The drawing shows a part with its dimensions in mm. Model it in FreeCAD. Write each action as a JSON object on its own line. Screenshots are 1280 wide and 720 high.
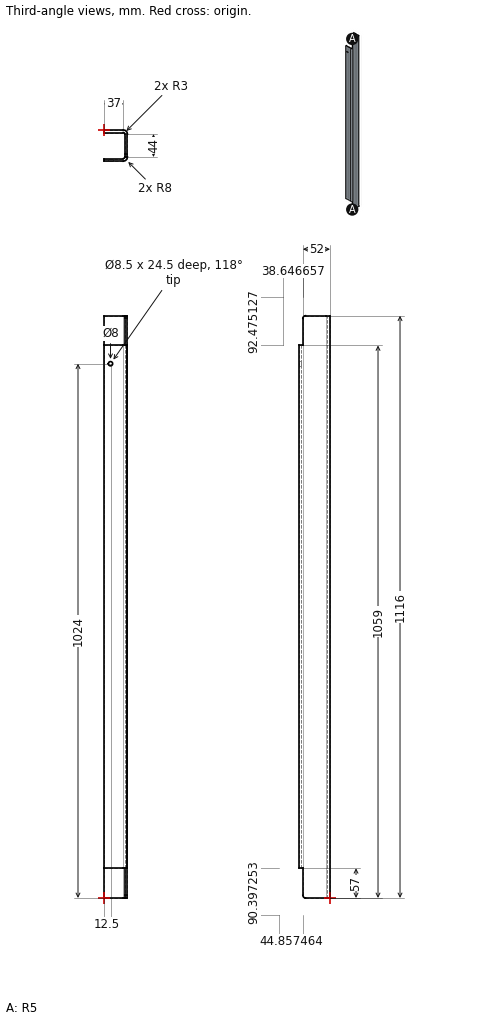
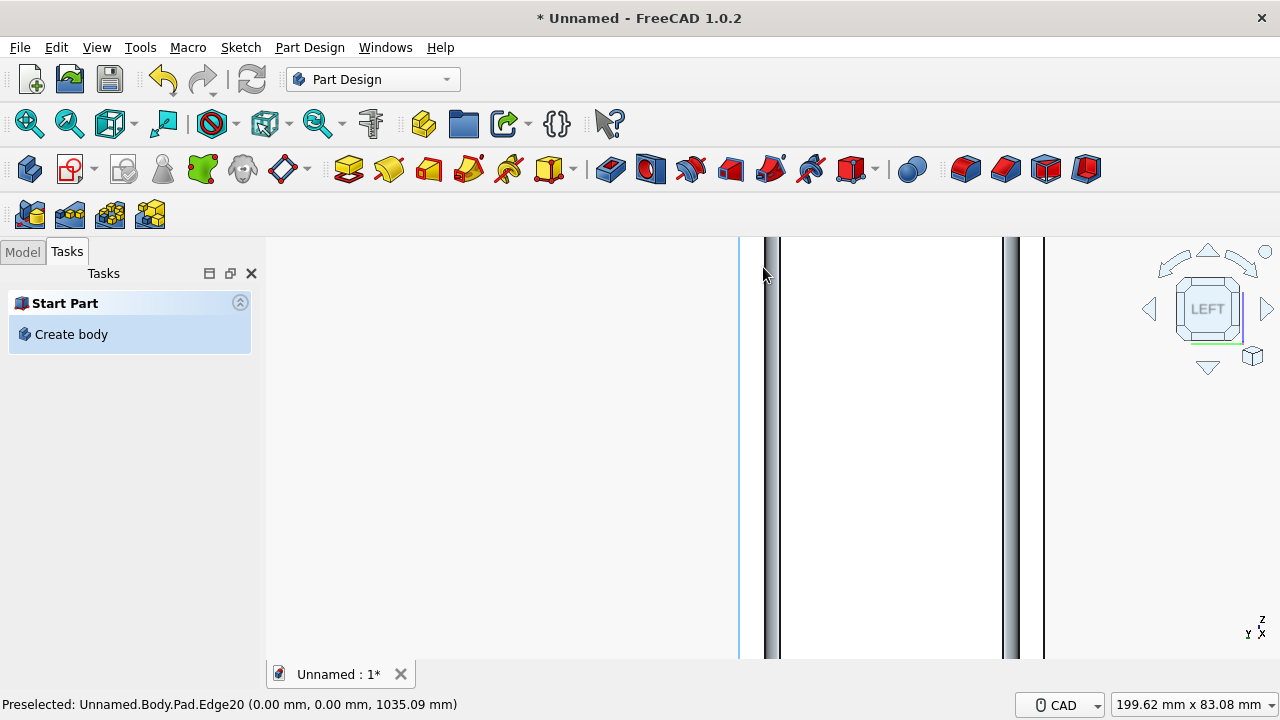
{"action": "left_click", "coordinate": [752, 273]}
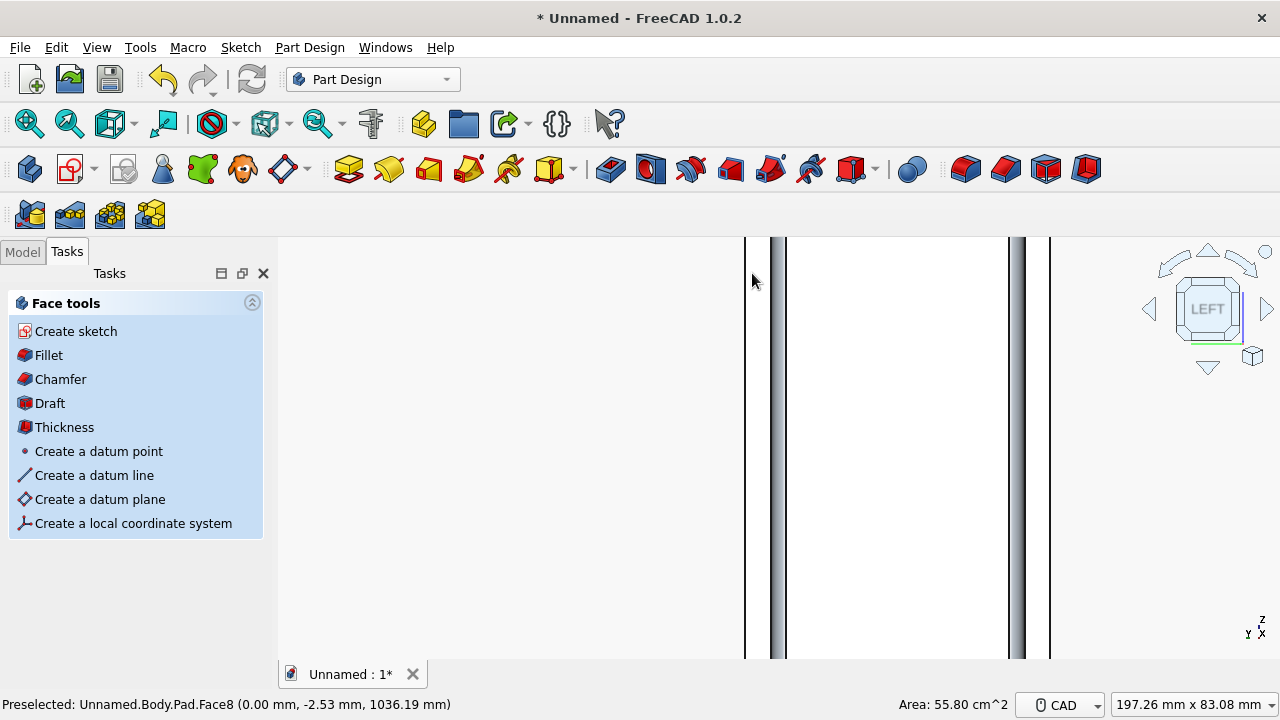
{"action": "left_click", "coordinate": [70, 170]}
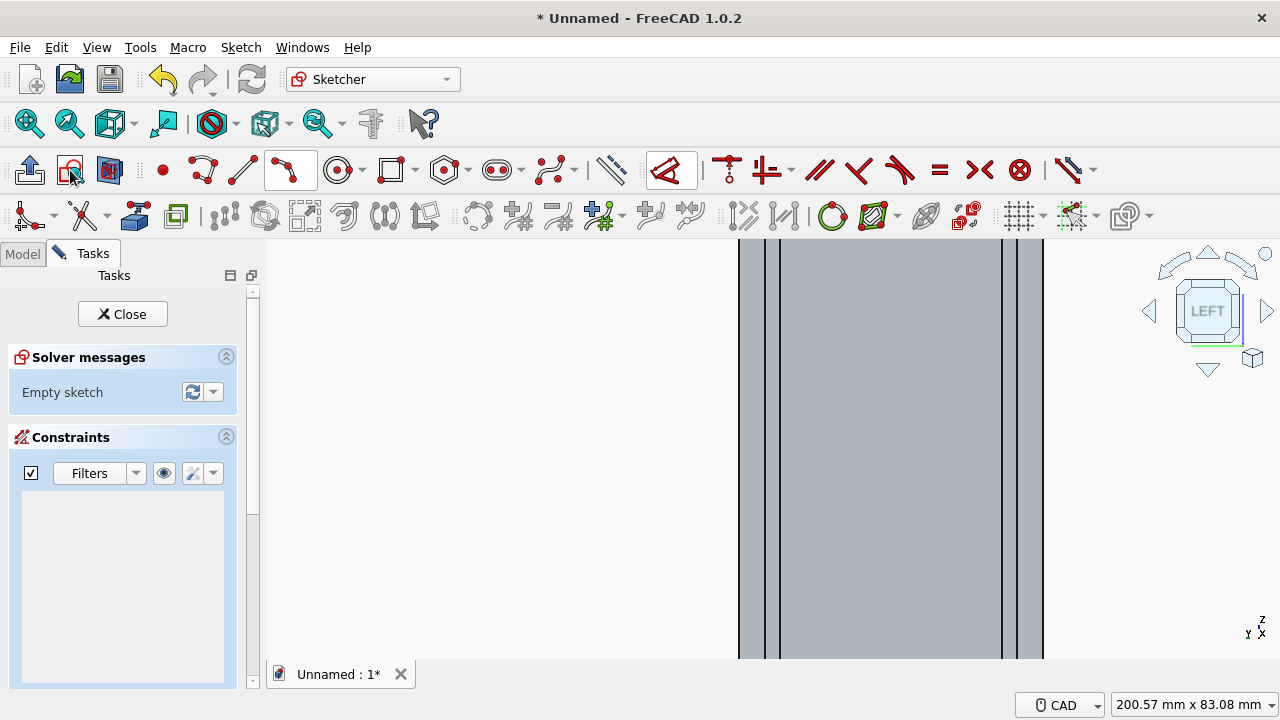
{"action": "scroll", "coordinate": [690, 332], "scroll_direction": "down", "scroll_amount": 15}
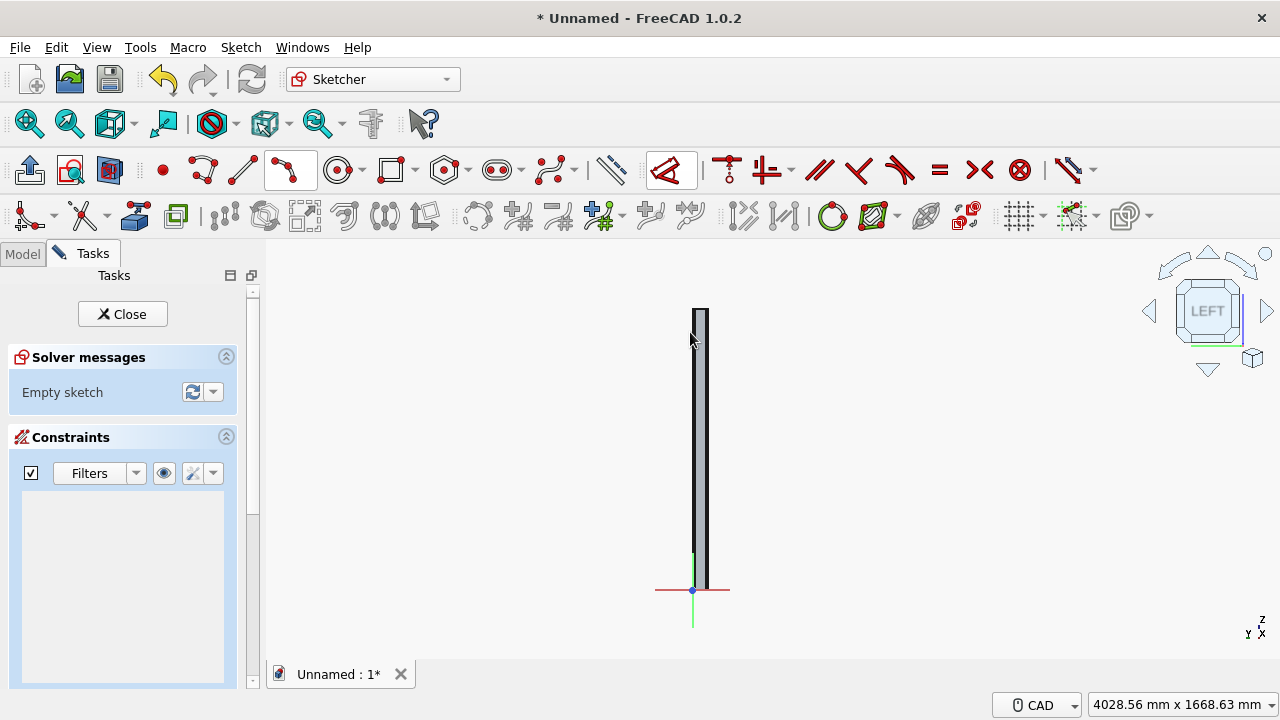
{"action": "left_click", "coordinate": [392, 170]}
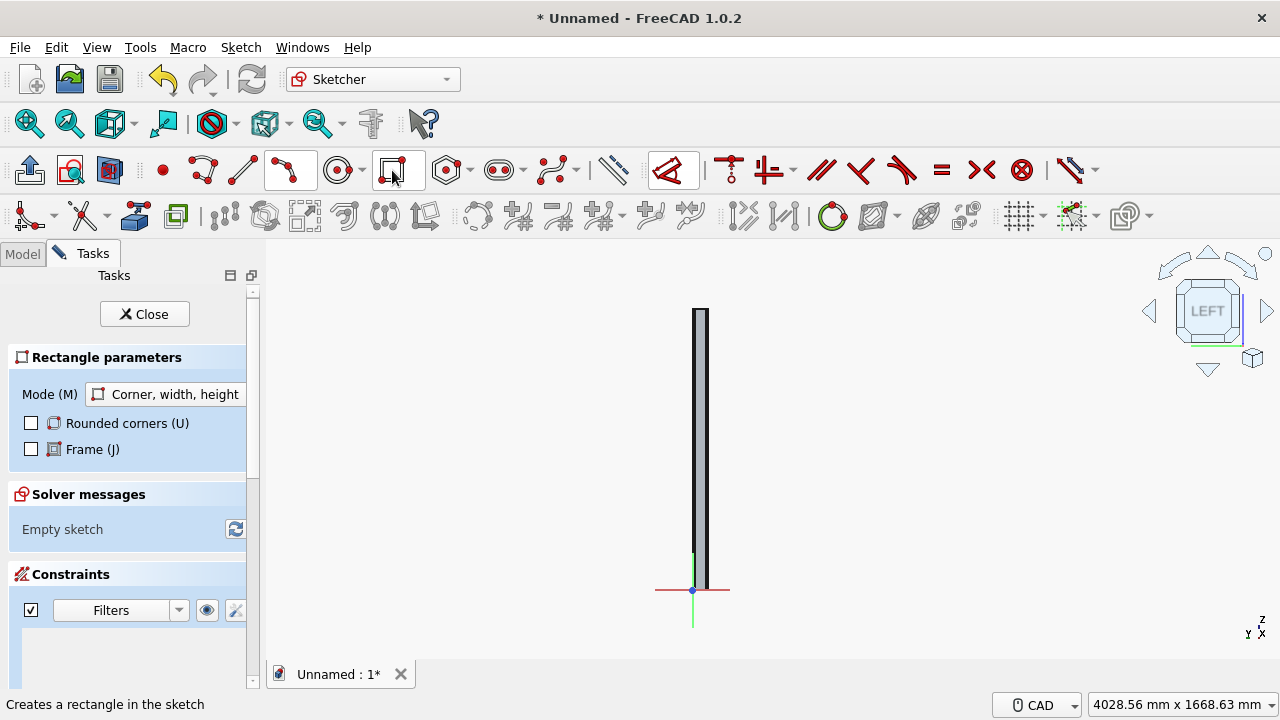
{"action": "scroll", "coordinate": [706, 300], "scroll_direction": "up", "scroll_amount": 3}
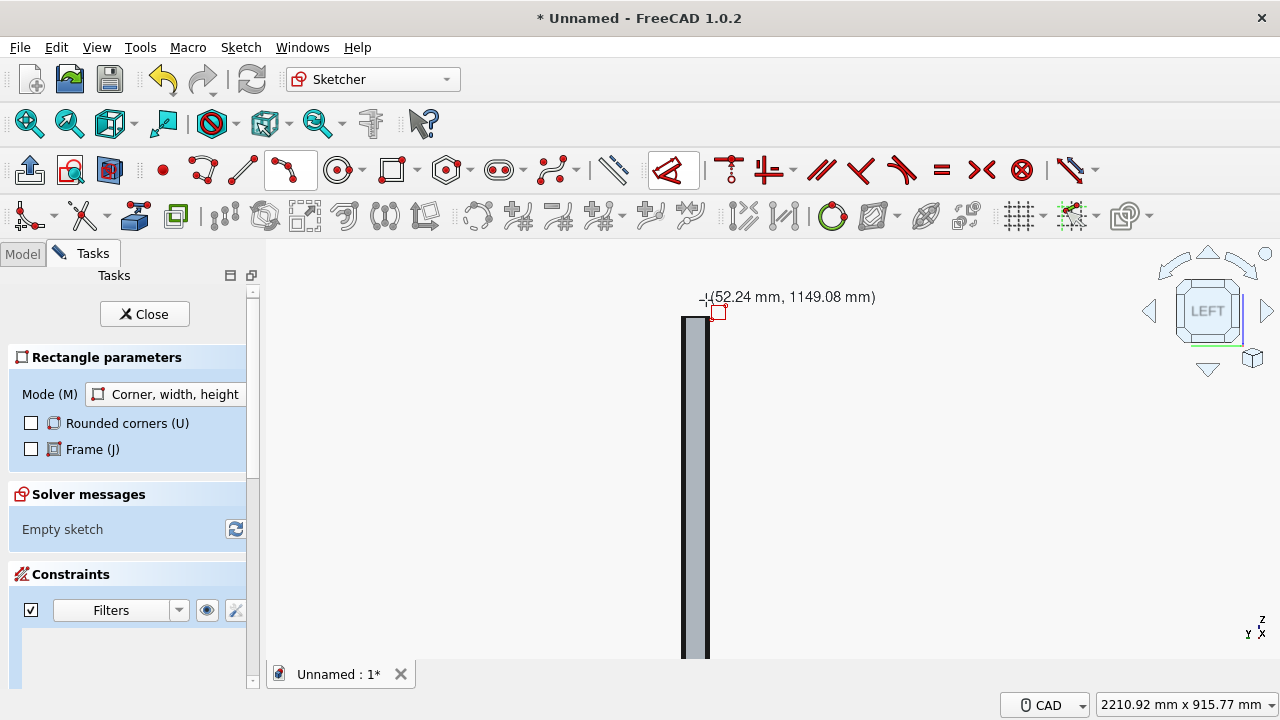
{"action": "left_click", "coordinate": [706, 301]}
{"action": "mouse_move", "coordinate": [723, 343]}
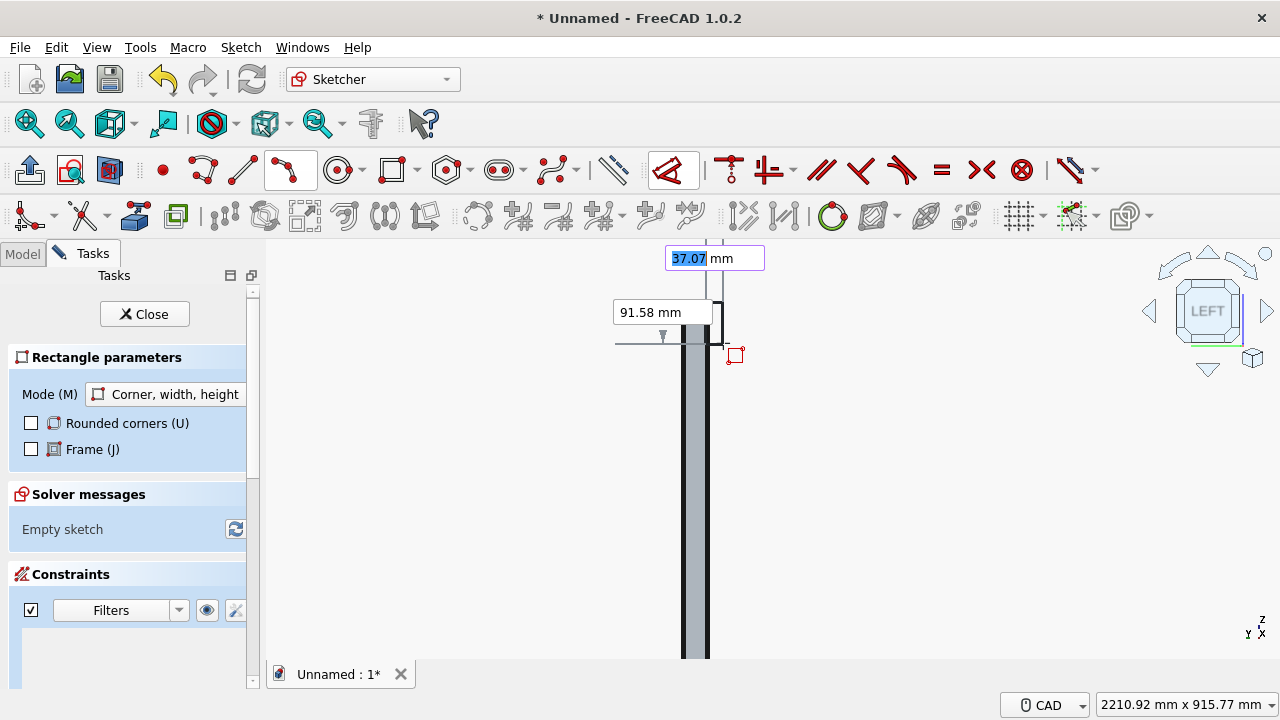
{"action": "type", "text": "38.646657"}
{"action": "key", "text": "Tab"}
{"action": "type", "text": "92.475127"}
{"action": "key", "text": "Return"}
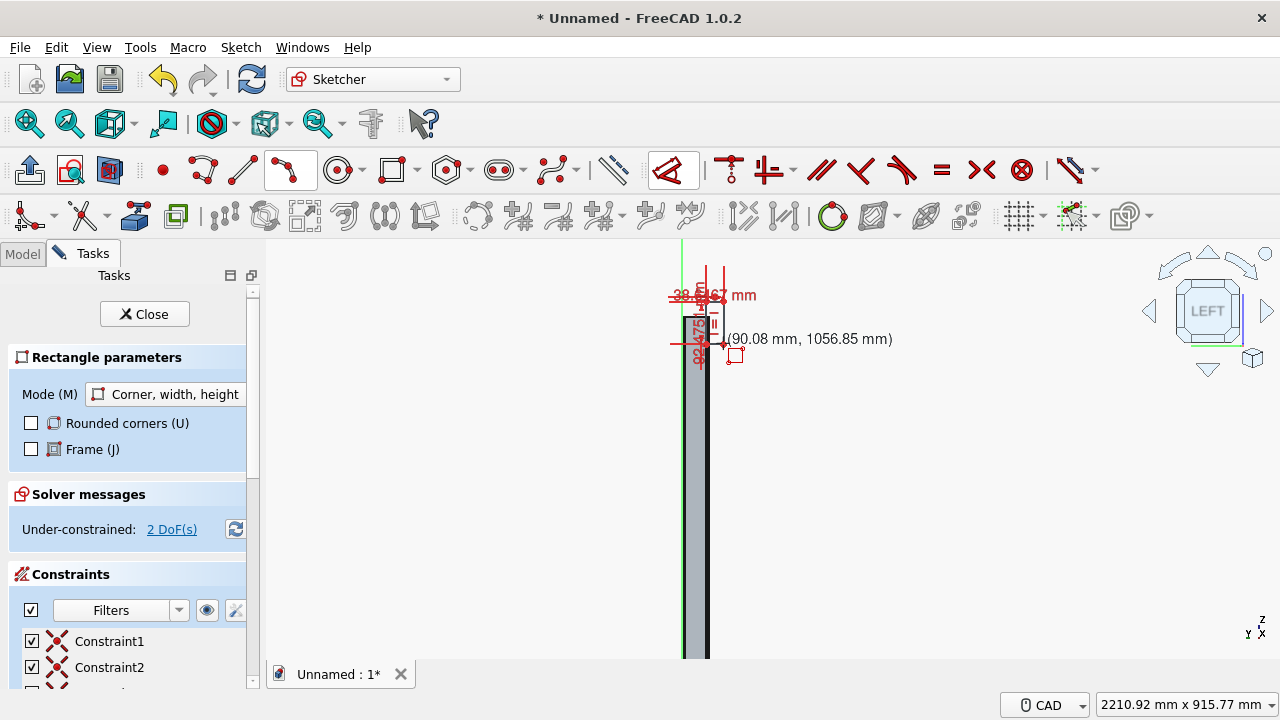
{"action": "scroll", "coordinate": [705, 348], "scroll_direction": "down", "scroll_amount": 4}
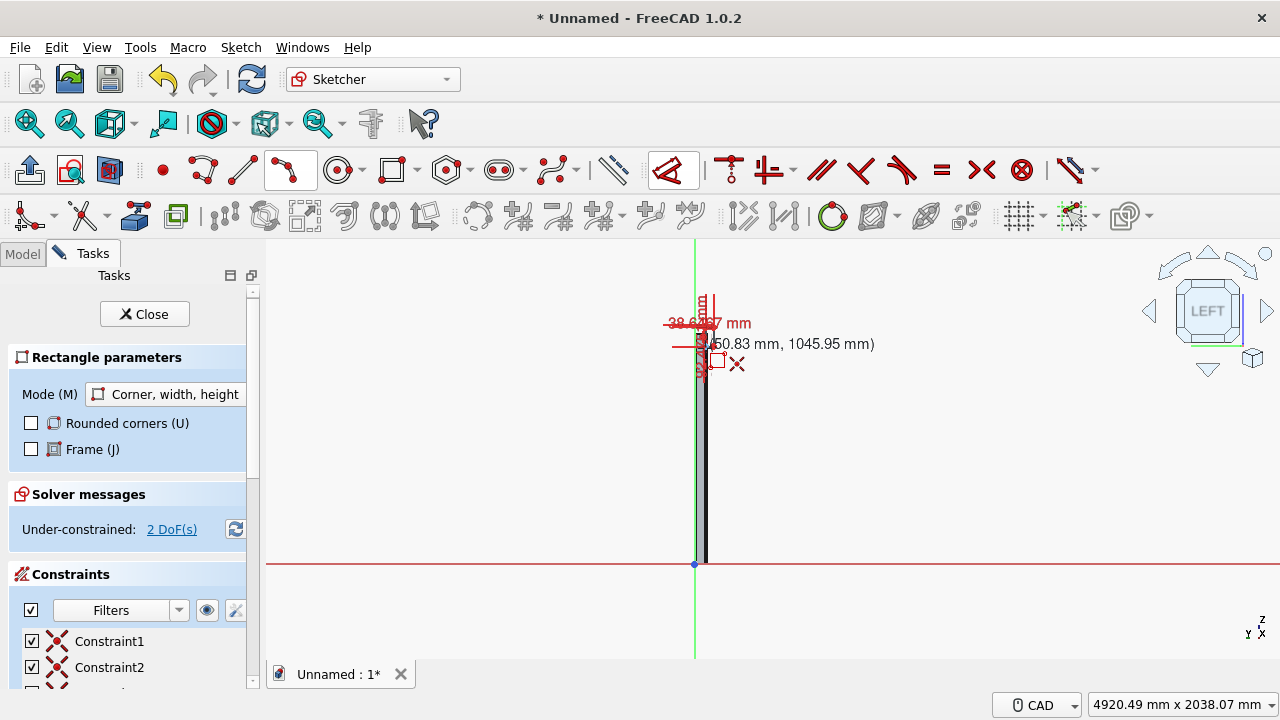
{"action": "scroll", "coordinate": [705, 552], "scroll_direction": "up", "scroll_amount": 3}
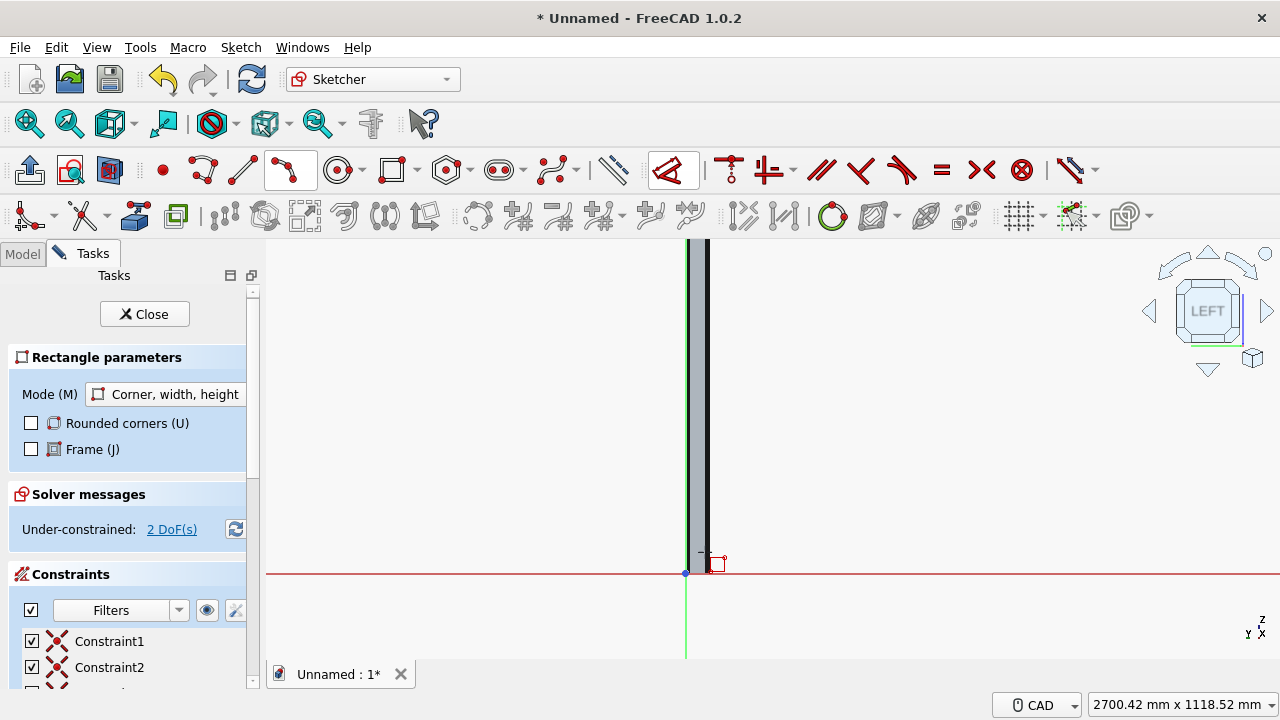
{"action": "left_click", "coordinate": [706, 552]}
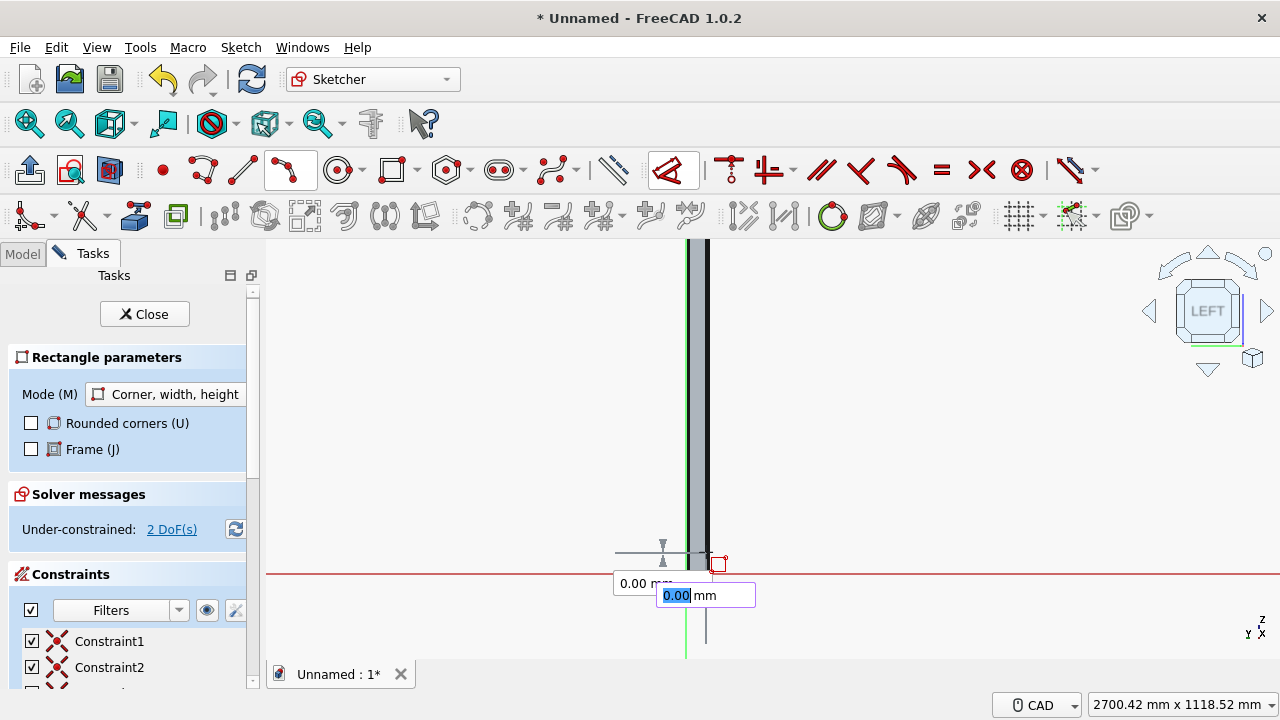
{"action": "scroll", "coordinate": [722, 586], "scroll_direction": "up", "scroll_amount": 2}
{"action": "mouse_move", "coordinate": [722, 586]}